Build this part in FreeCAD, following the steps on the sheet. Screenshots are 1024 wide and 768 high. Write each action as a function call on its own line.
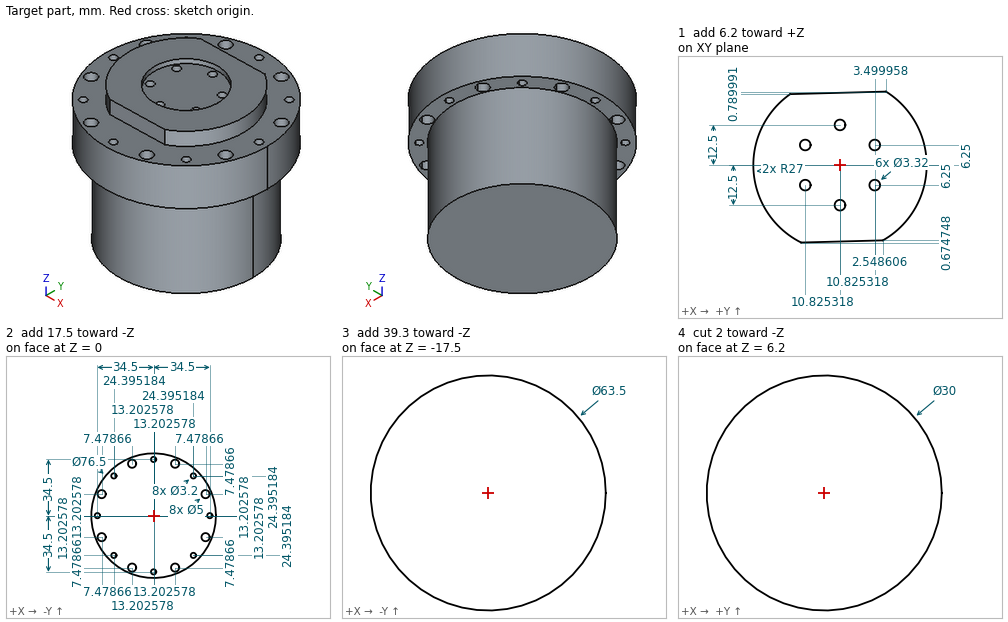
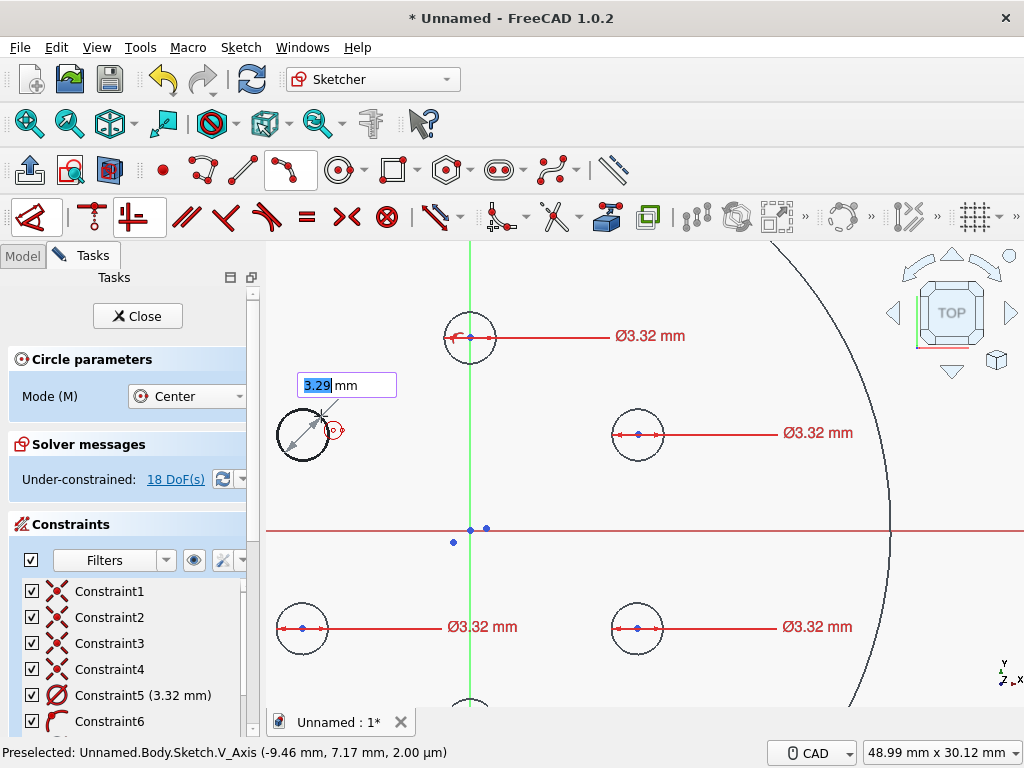
text(3.32)
key(Return)
key(Escape)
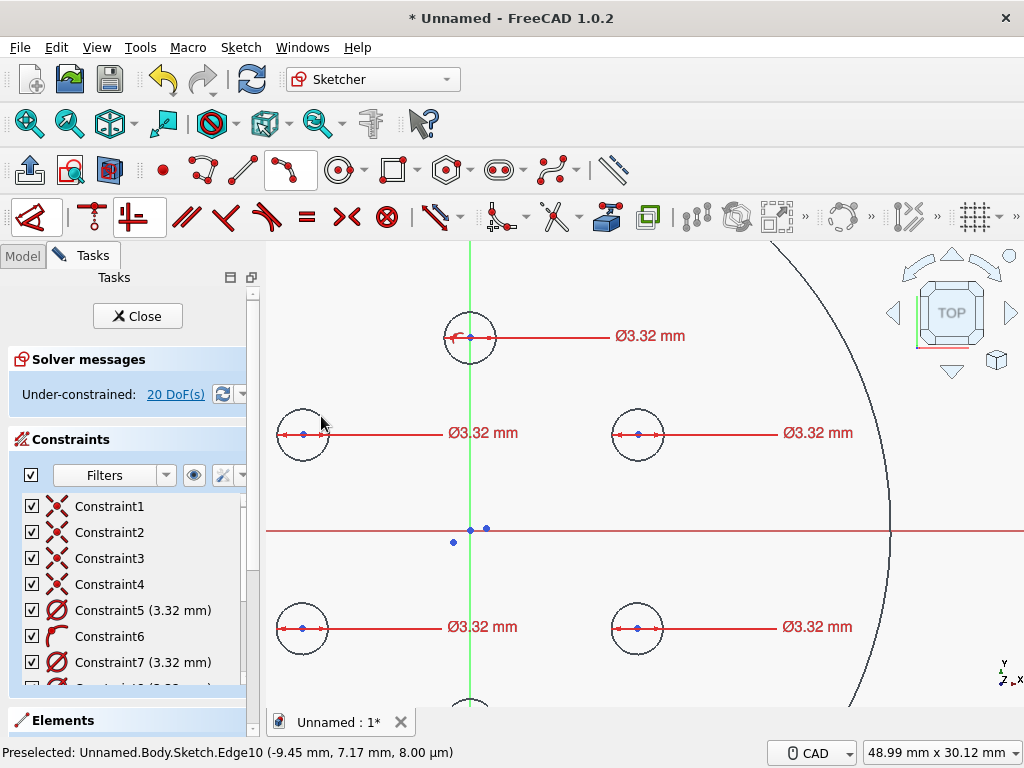
scroll(638, 435, down, 5)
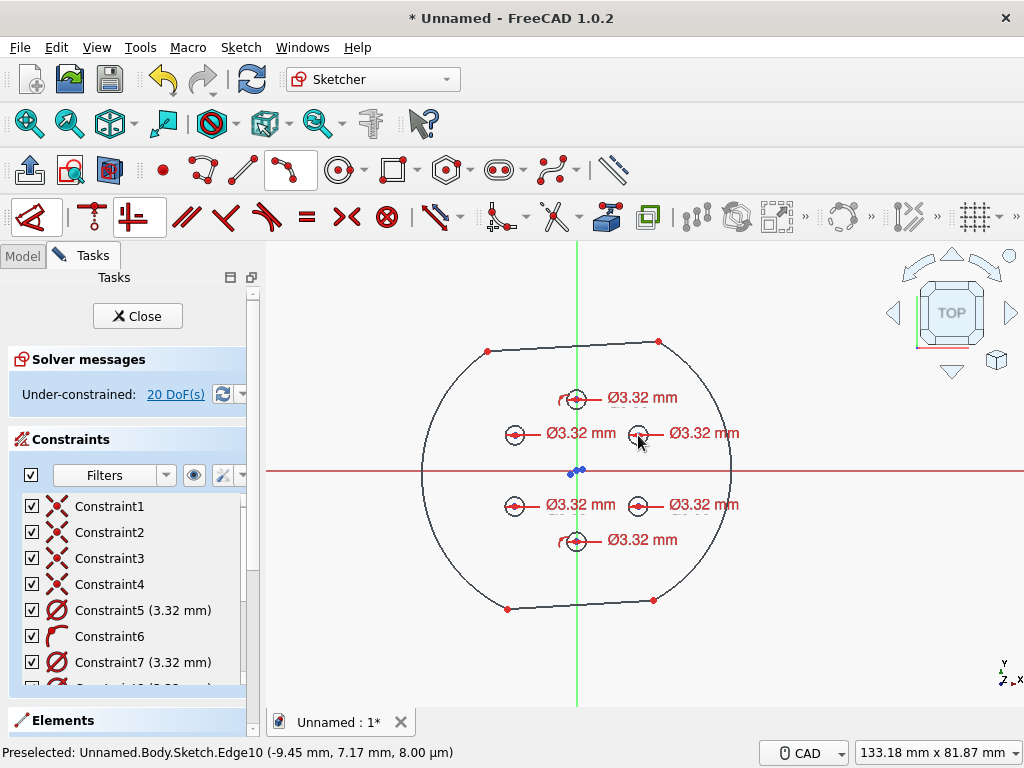
click(431, 424)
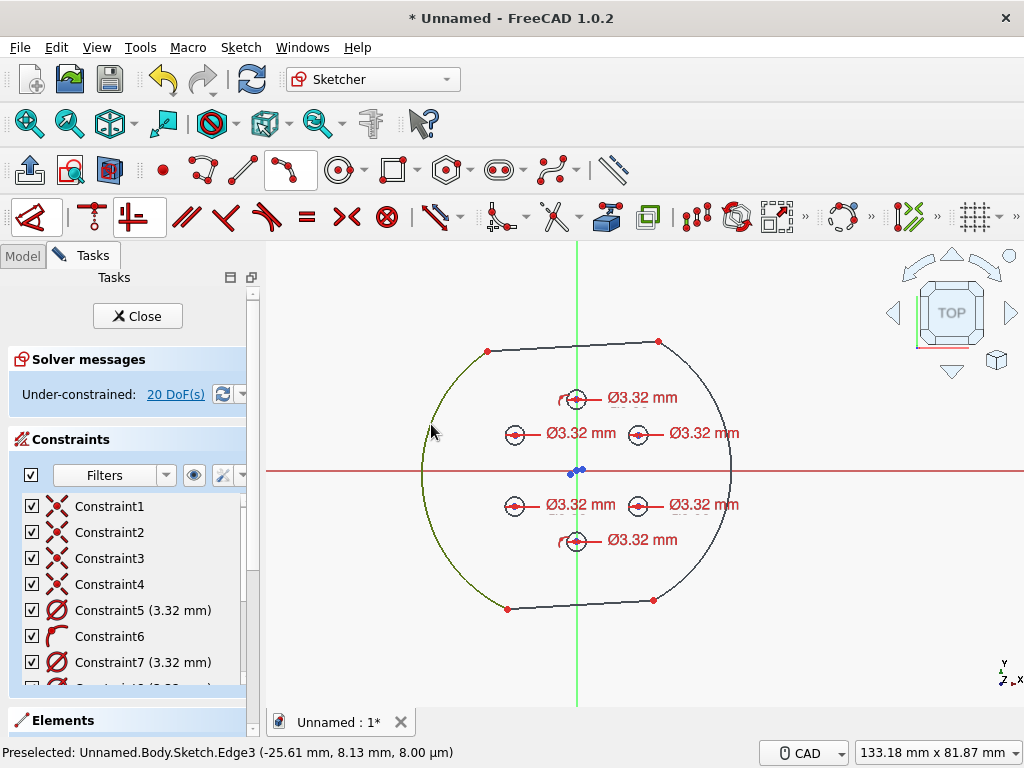
click(717, 533)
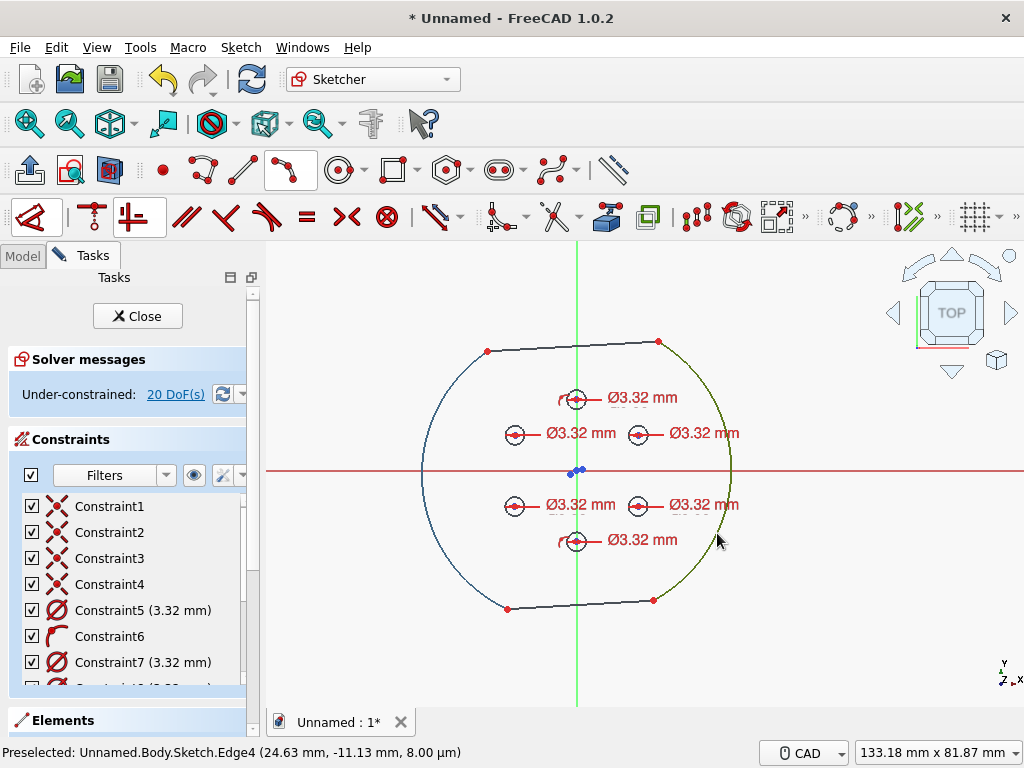
click(92, 218)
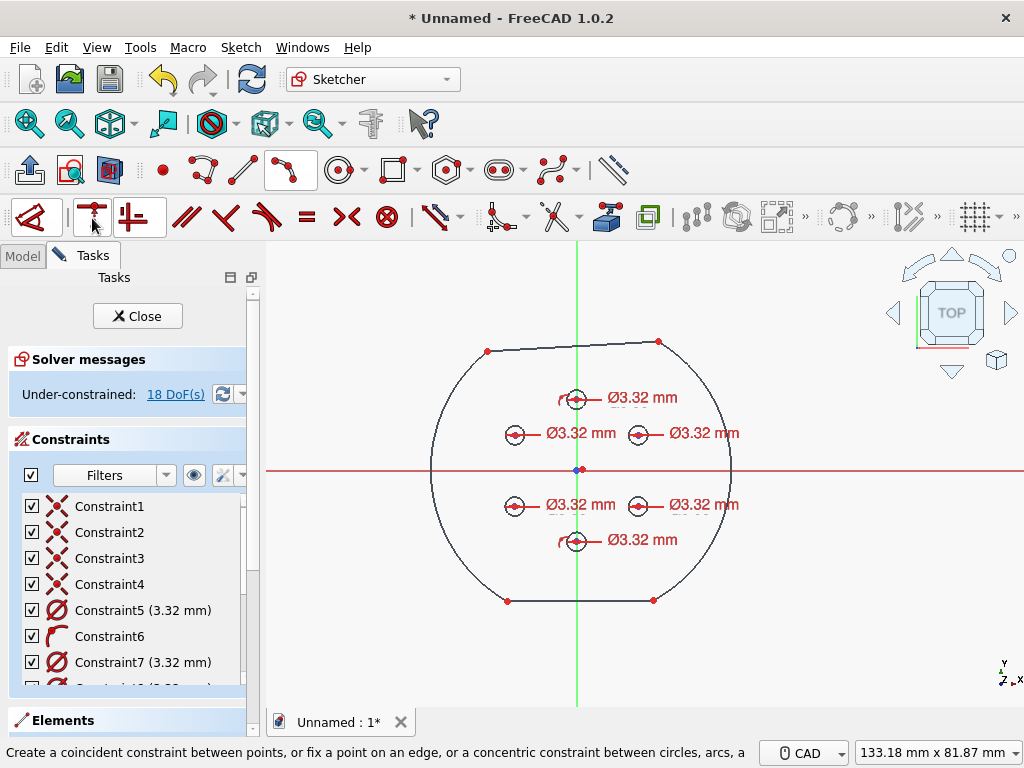
scroll(579, 470, up, 8)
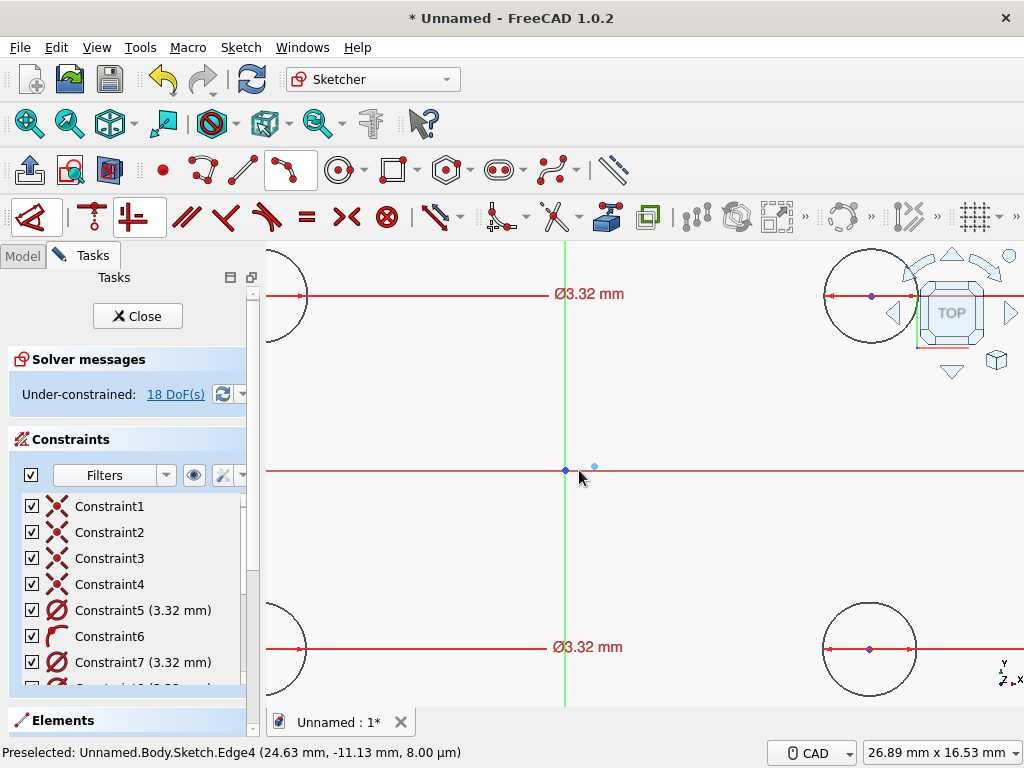
drag(555, 457, 604, 481)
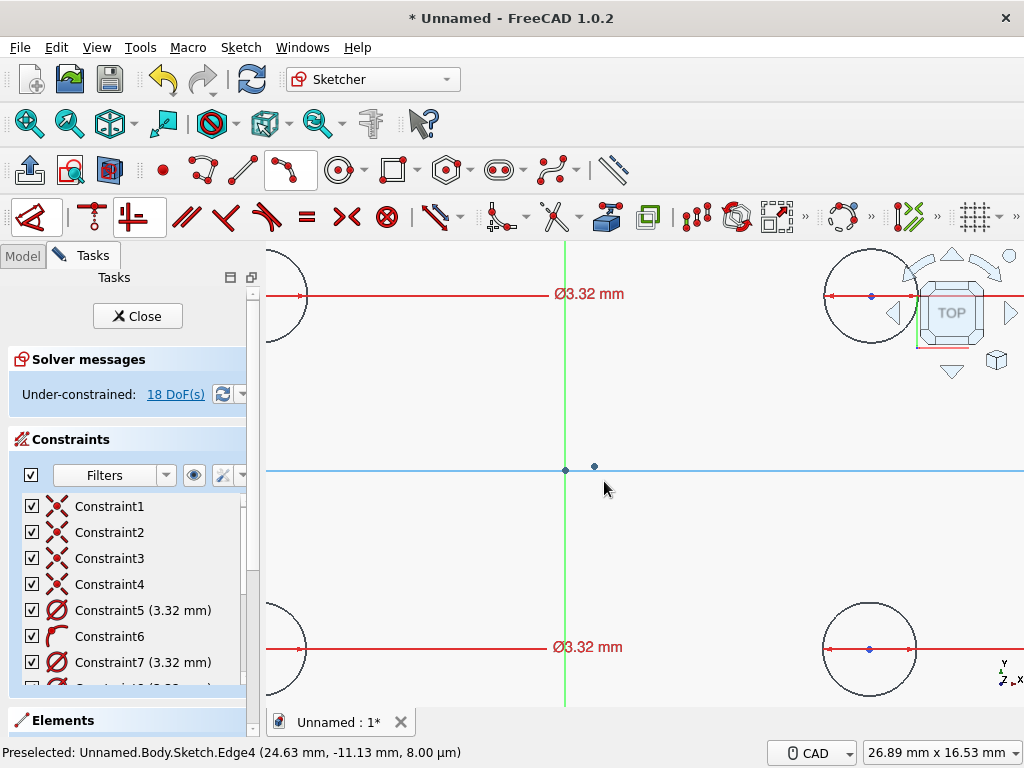
click(92, 218)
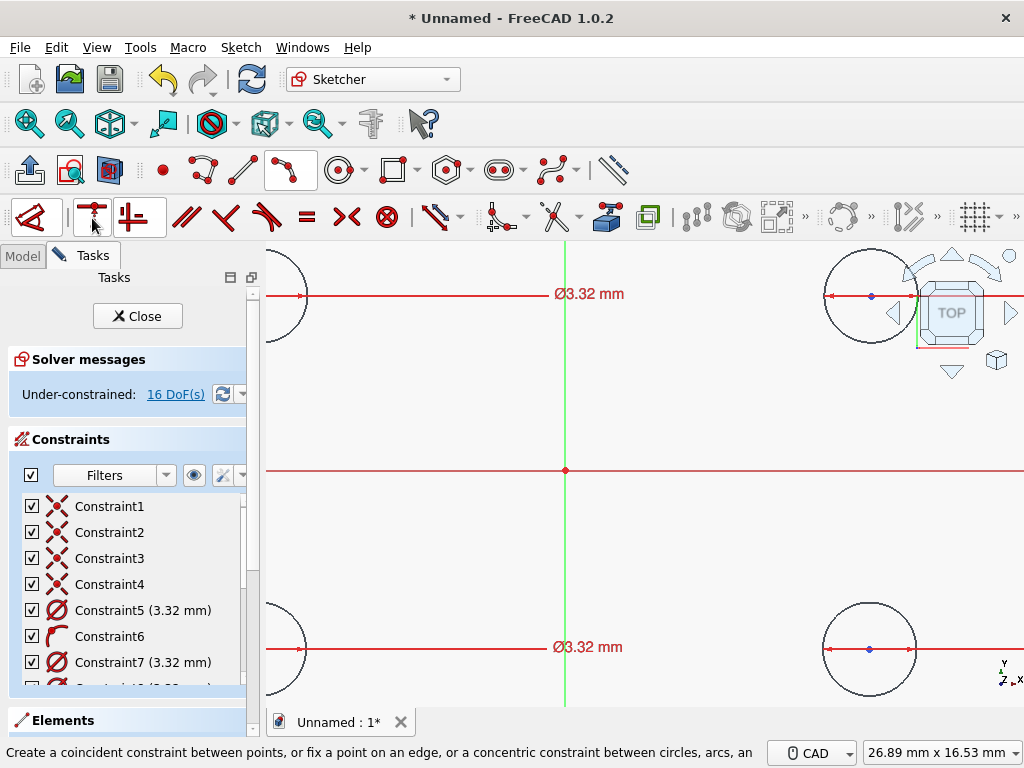
scroll(579, 470, down, 8)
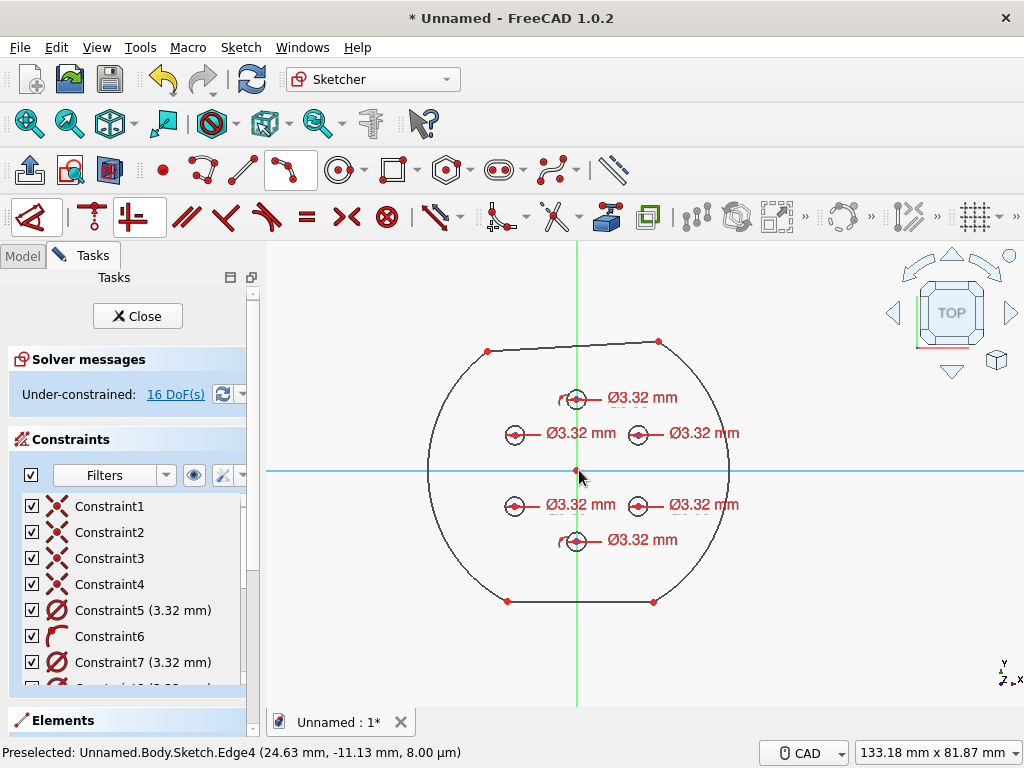
click(436, 423)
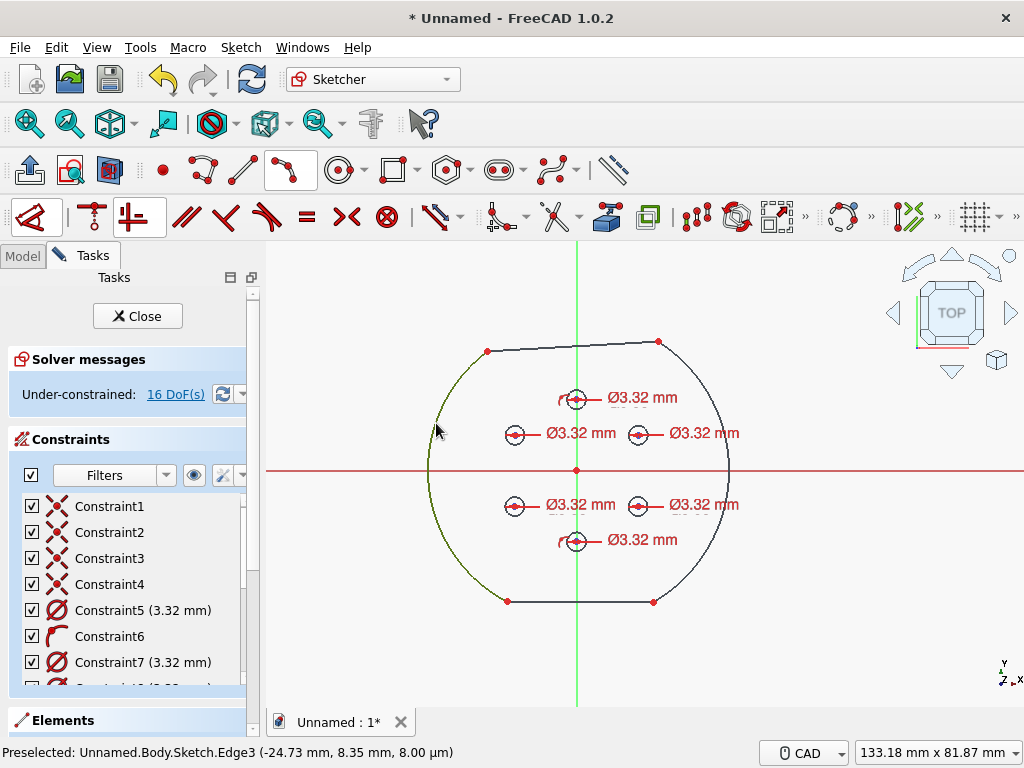
click(715, 534)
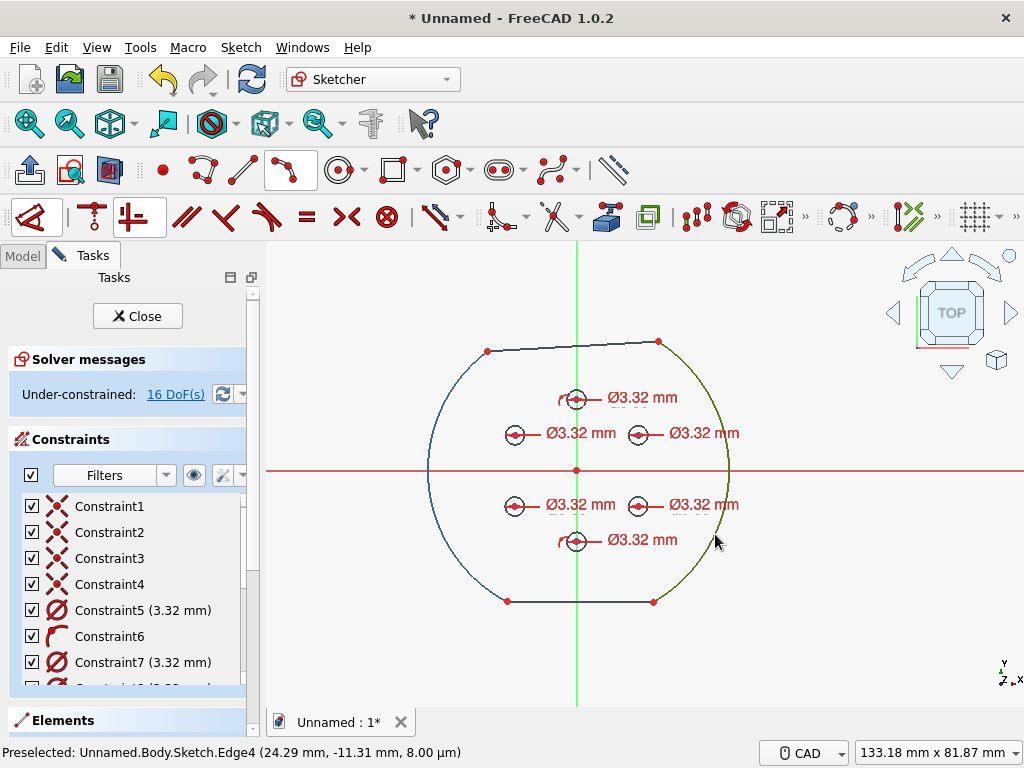
click(308, 218)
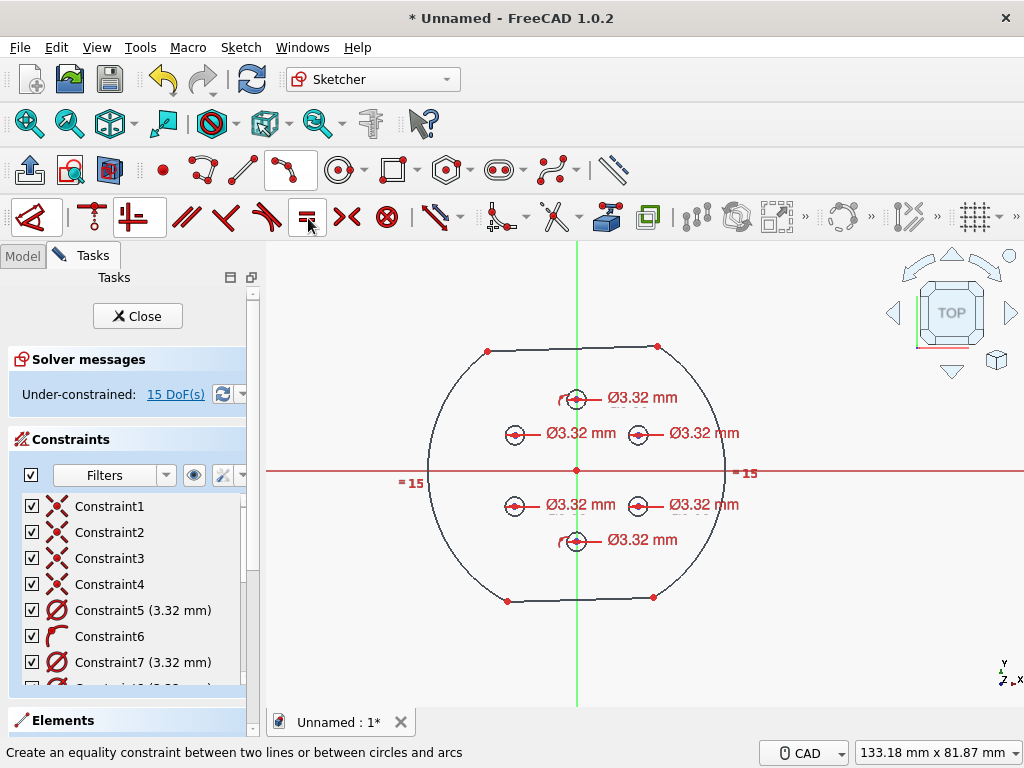
click(638, 507)